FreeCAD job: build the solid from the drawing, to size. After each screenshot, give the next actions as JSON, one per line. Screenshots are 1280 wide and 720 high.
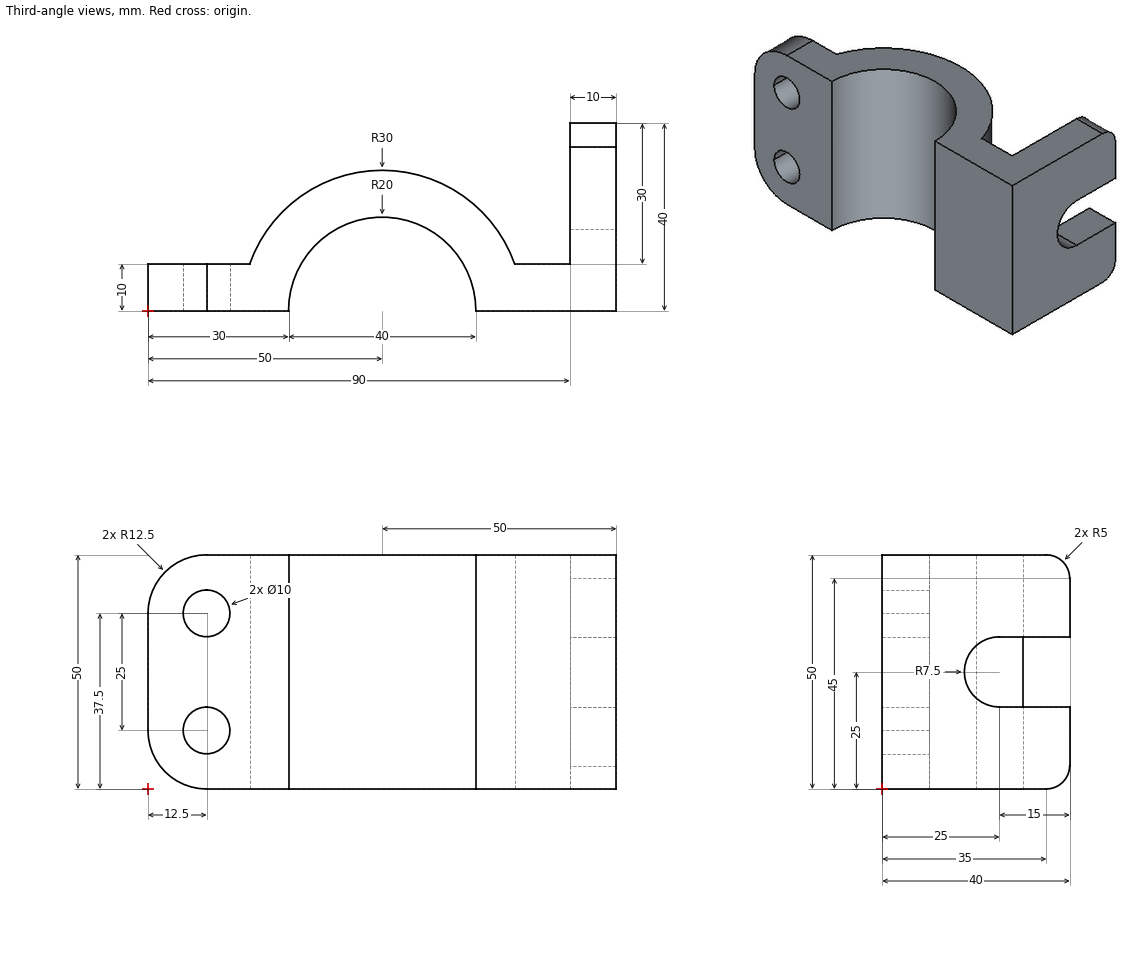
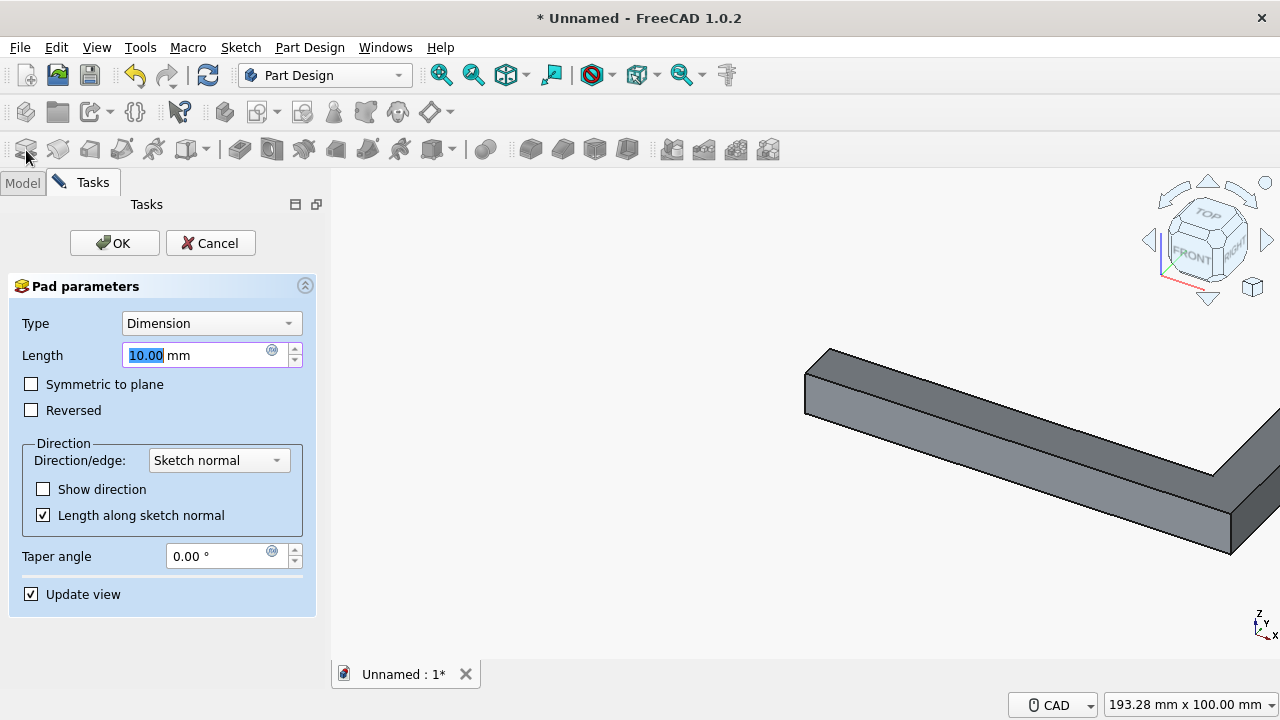
{"action": "type", "text": "50"}
{"action": "key", "text": "Tab"}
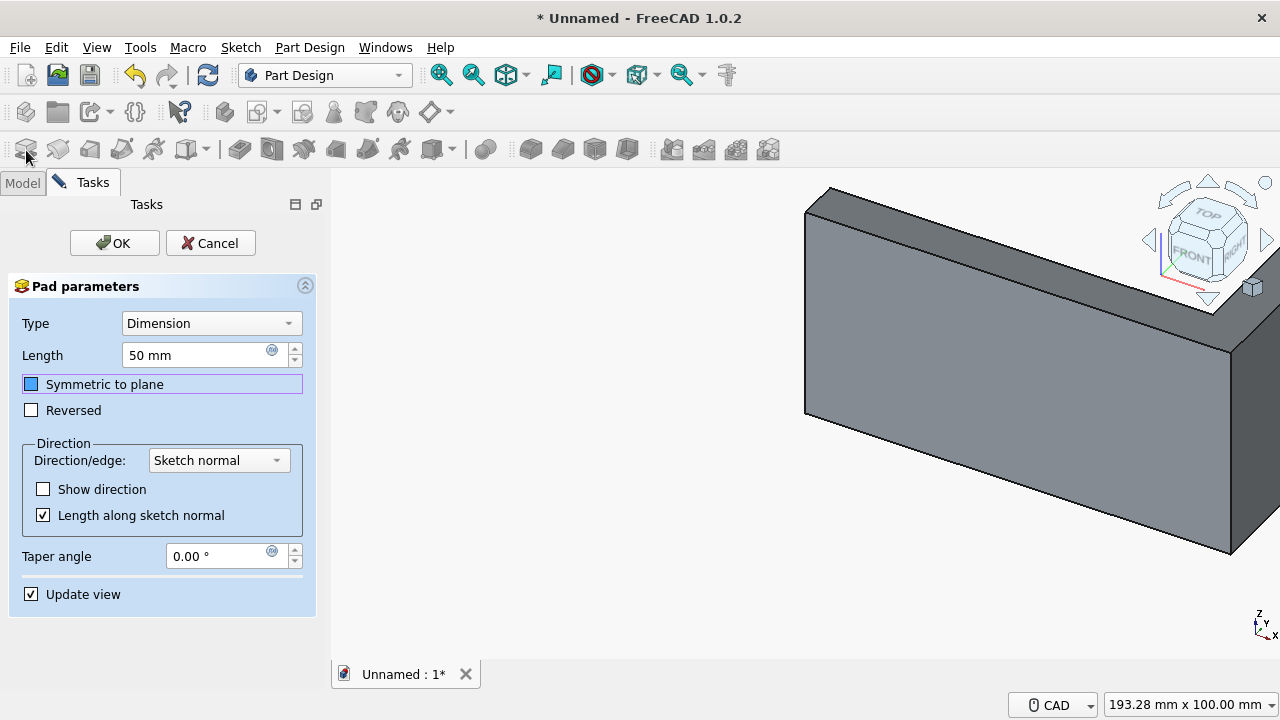
{"action": "left_click", "coordinate": [115, 243]}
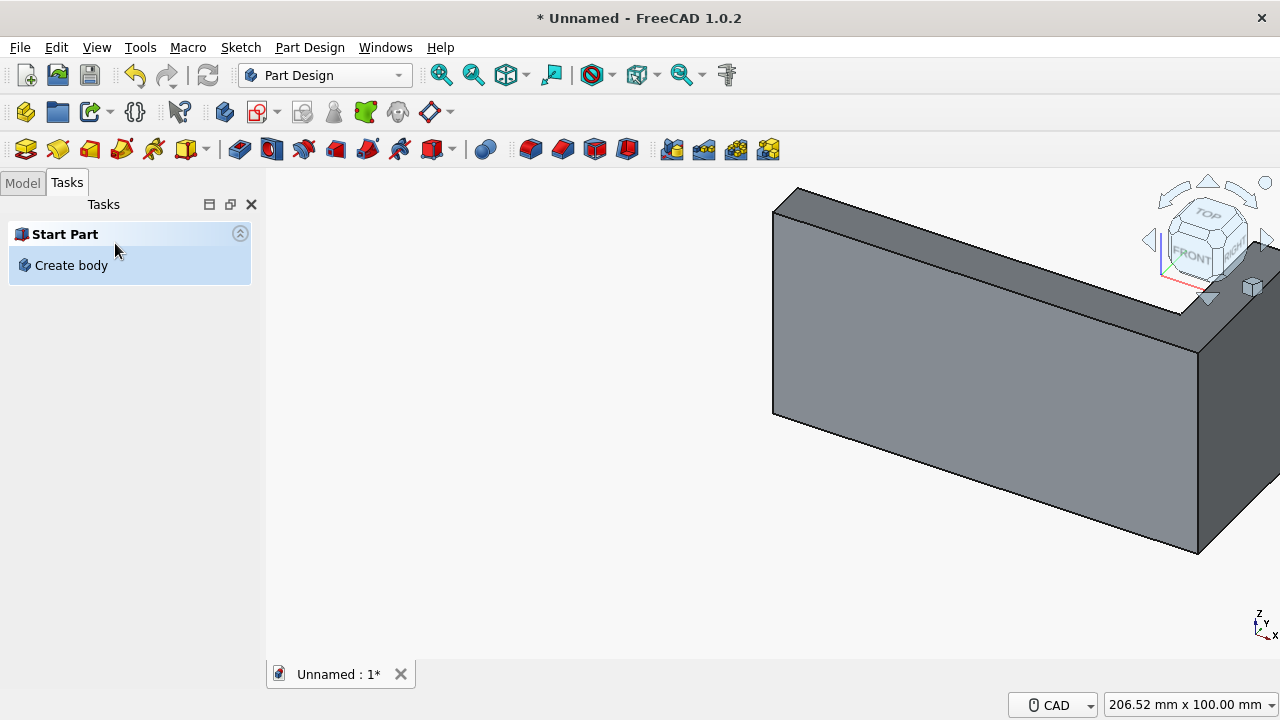
{"action": "left_click", "coordinate": [442, 76]}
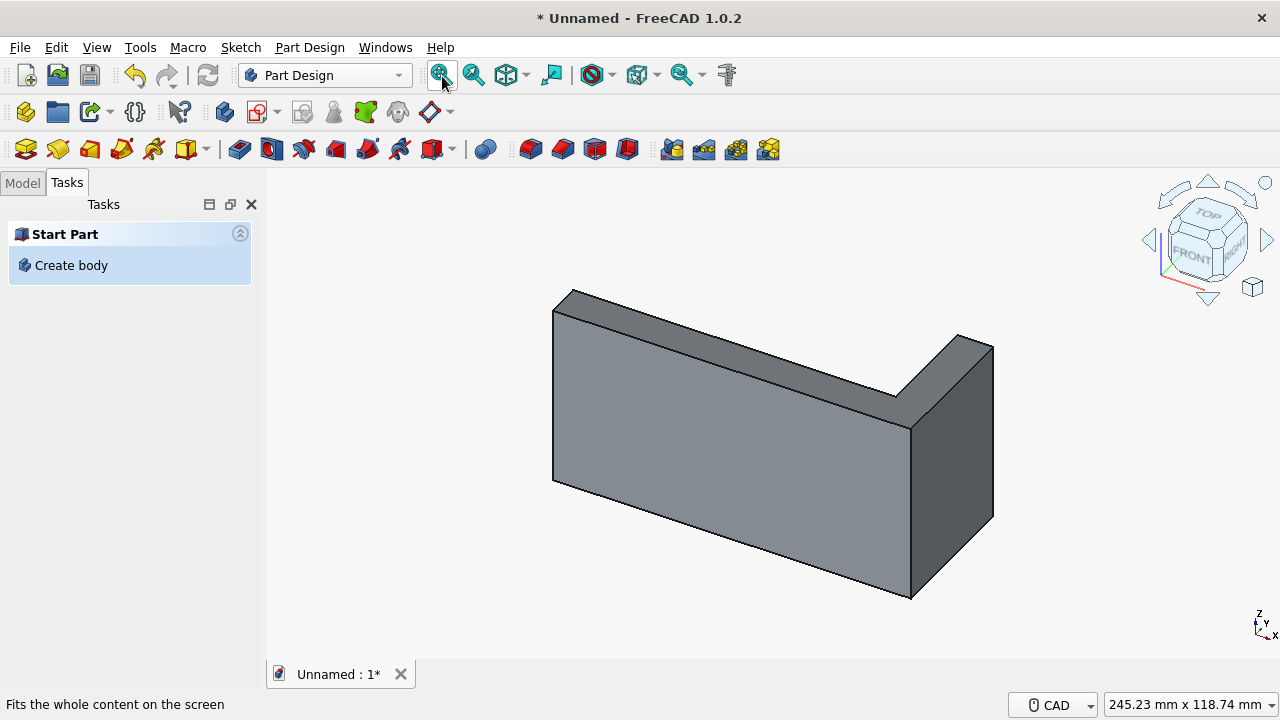
{"action": "left_click", "coordinate": [952, 472]}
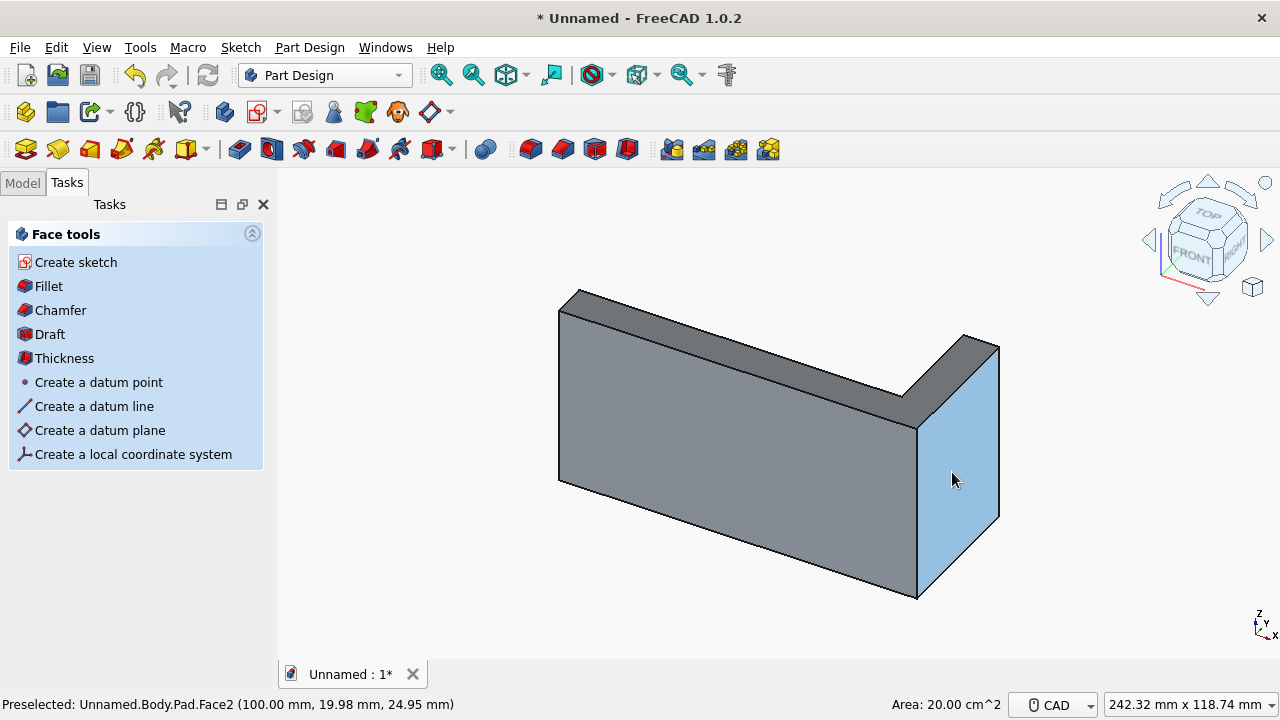
{"action": "left_click", "coordinate": [258, 112]}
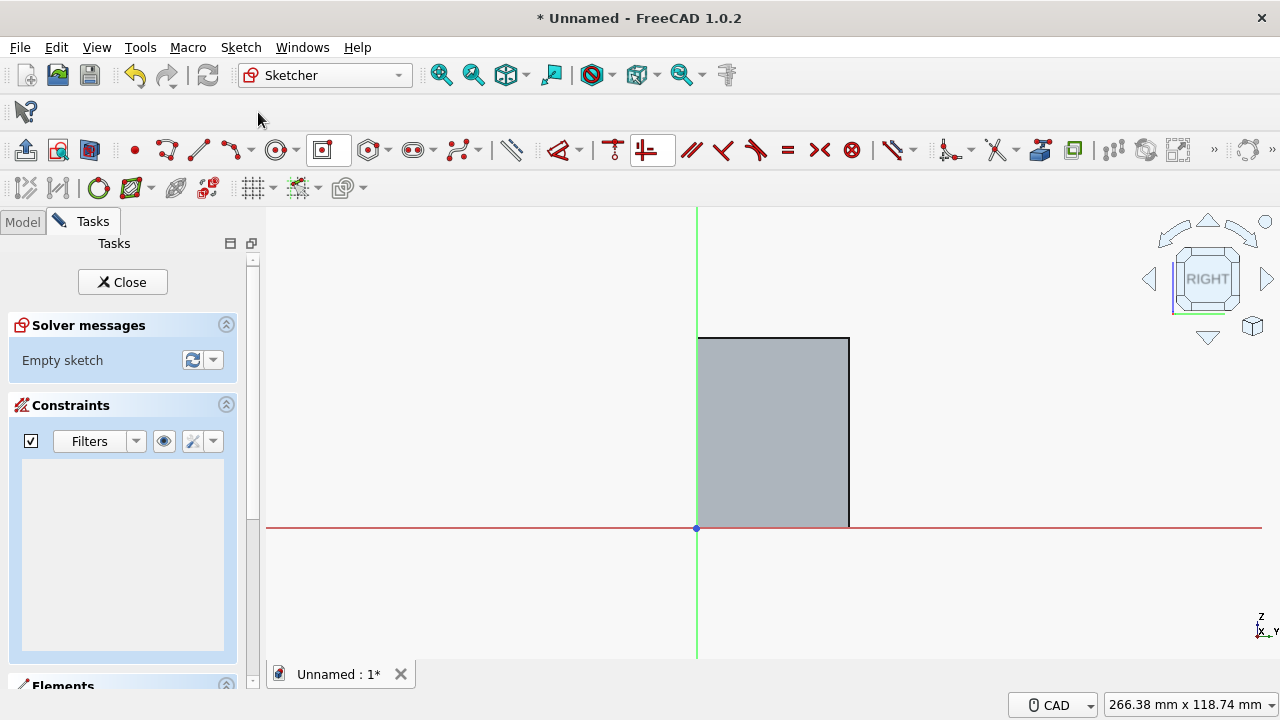
{"action": "scroll", "coordinate": [912, 433], "scroll_direction": "up", "scroll_amount": 2}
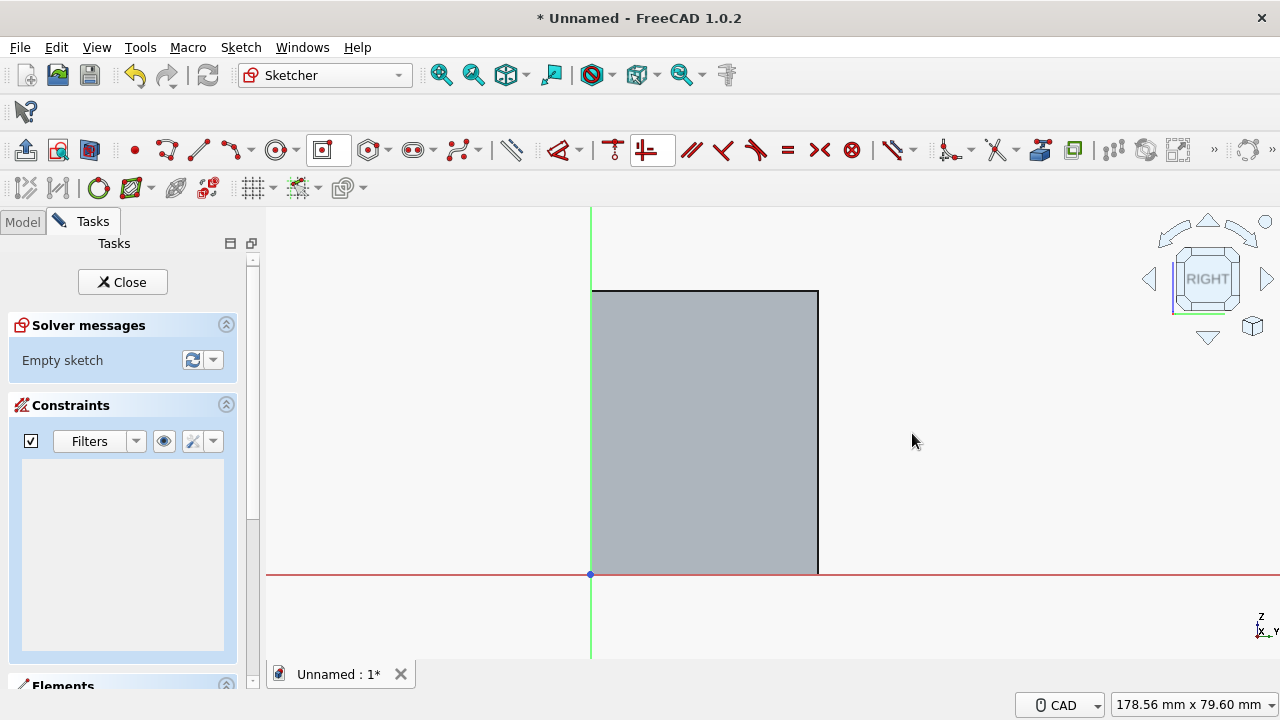
{"action": "left_click", "coordinate": [168, 150]}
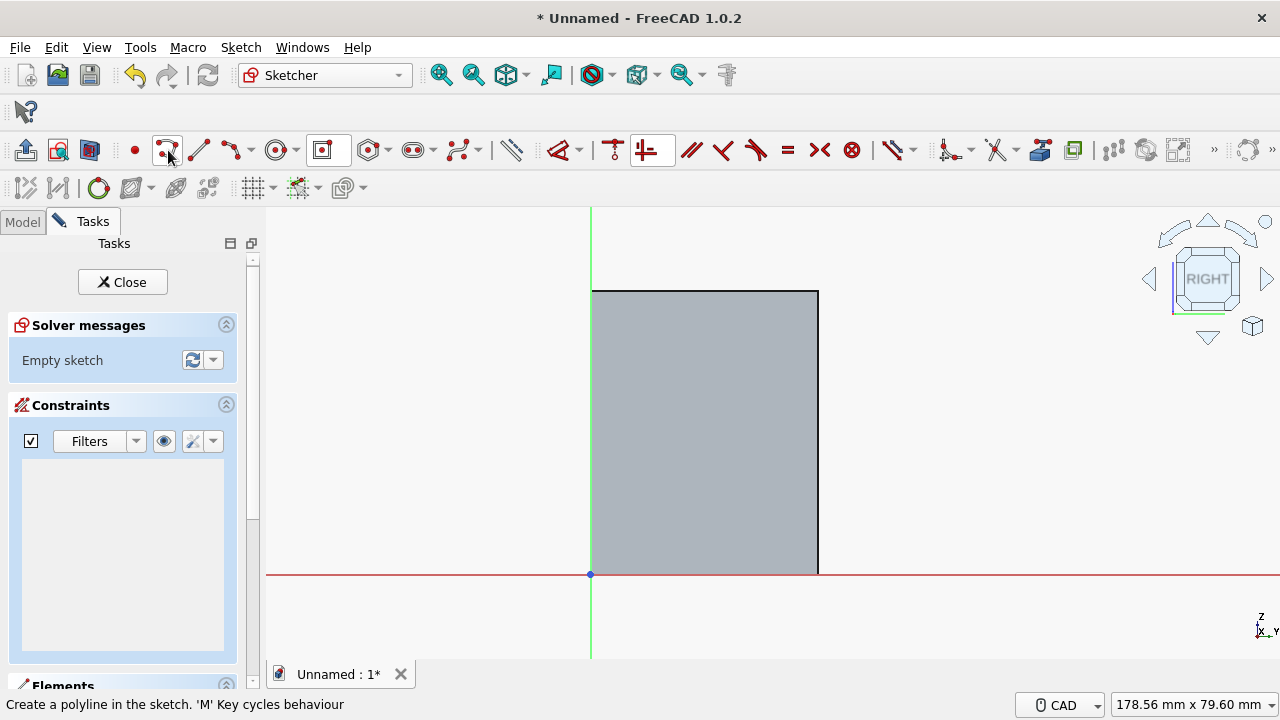
{"action": "left_click", "coordinate": [818, 319]}
{"action": "left_click", "coordinate": [818, 291]}
{"action": "left_click", "coordinate": [790, 291]}
{"action": "right_click", "coordinate": [790, 291]}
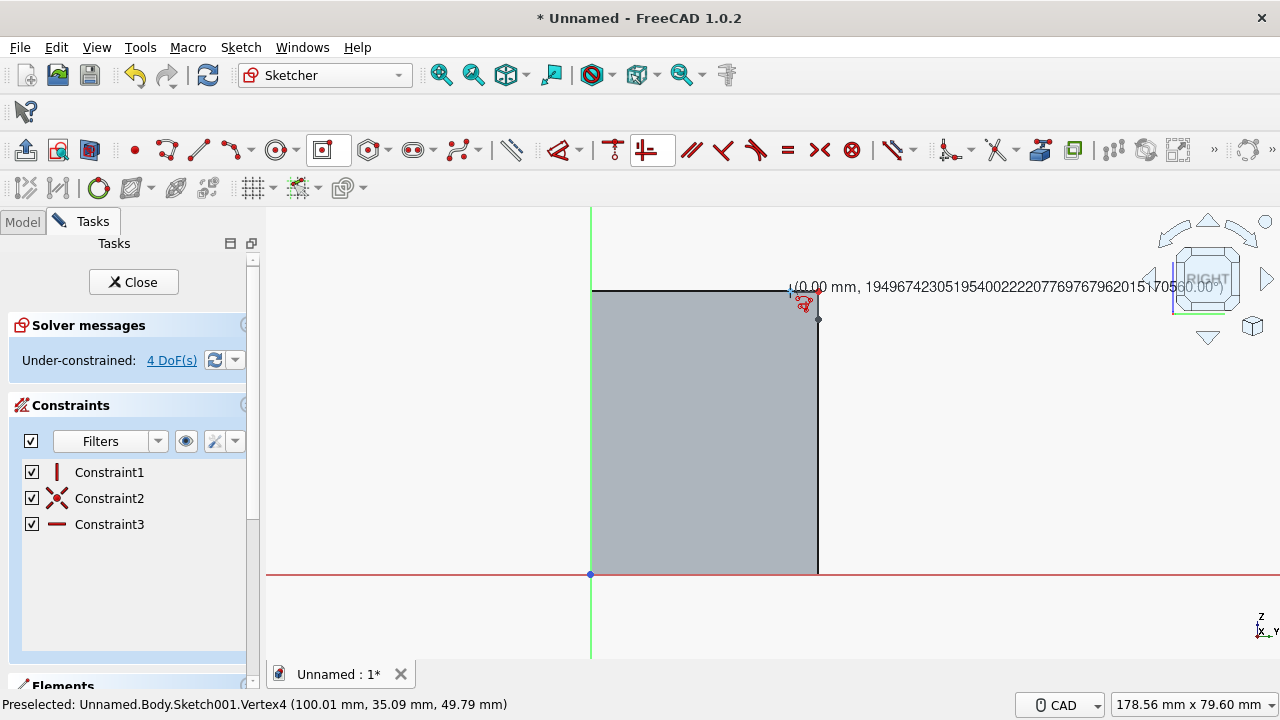
{"action": "left_click", "coordinate": [232, 150]}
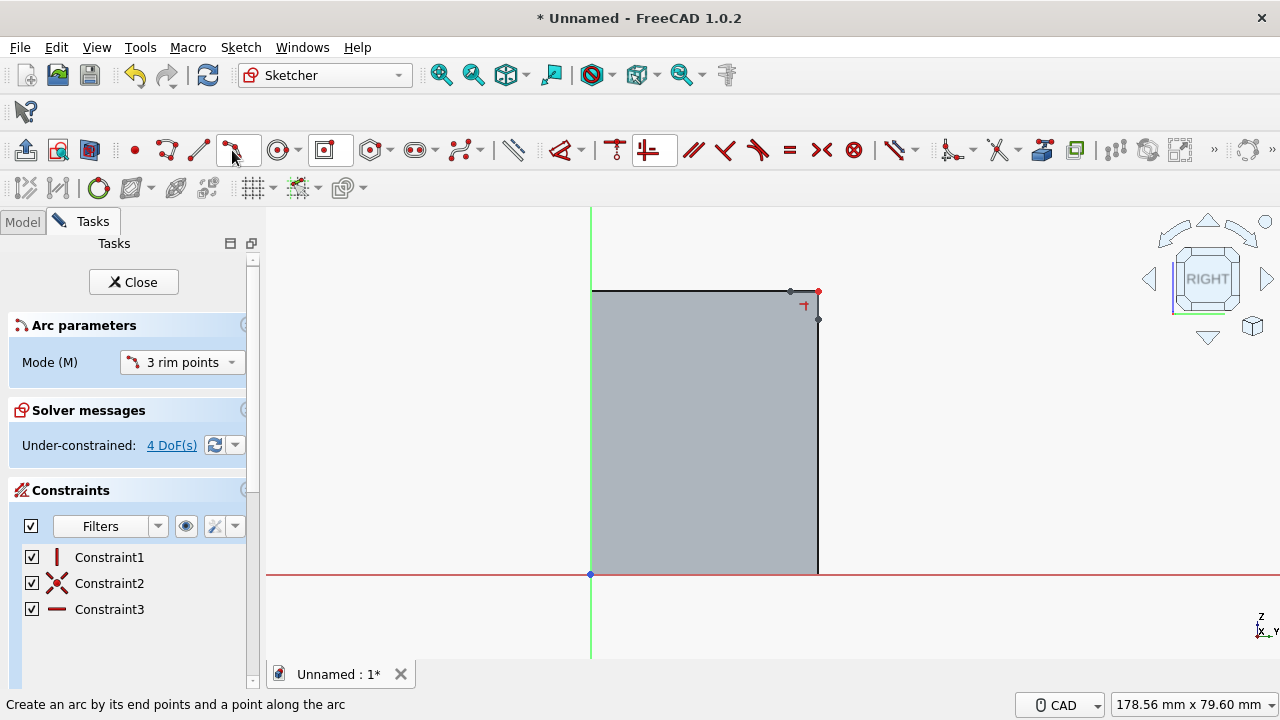
{"action": "left_click", "coordinate": [790, 292]}
{"action": "left_click", "coordinate": [818, 320]}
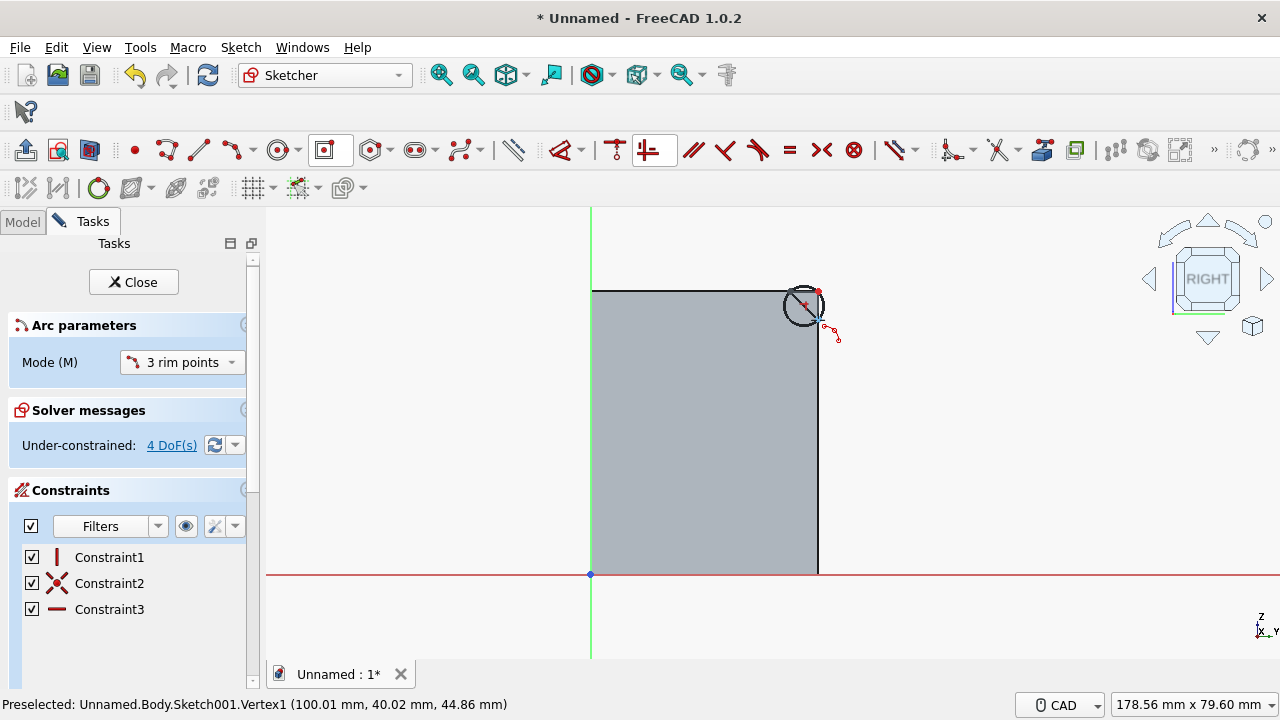
{"action": "scroll", "coordinate": [810, 299], "scroll_direction": "up", "scroll_amount": 4}